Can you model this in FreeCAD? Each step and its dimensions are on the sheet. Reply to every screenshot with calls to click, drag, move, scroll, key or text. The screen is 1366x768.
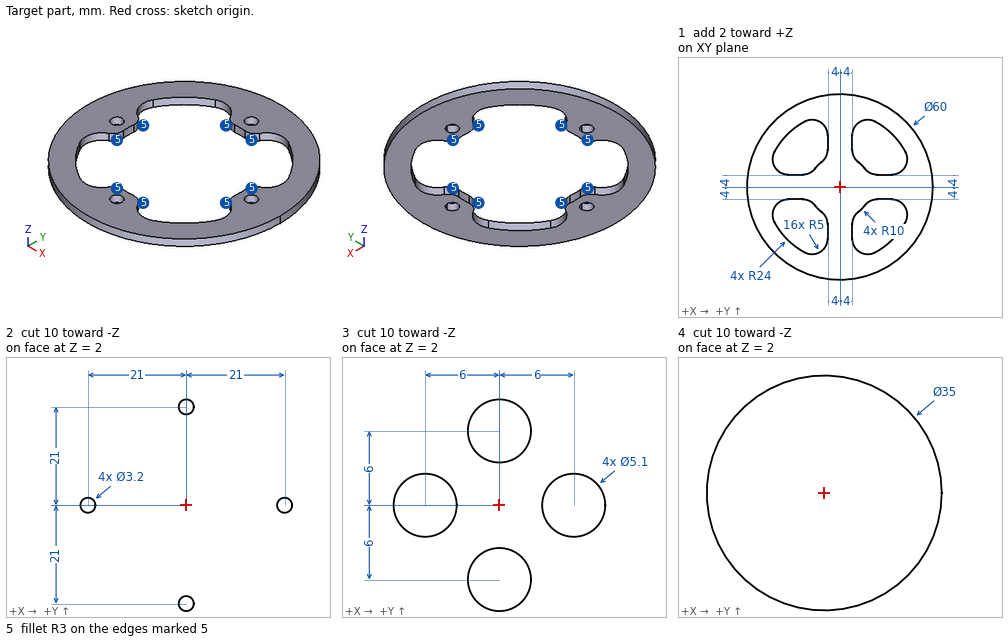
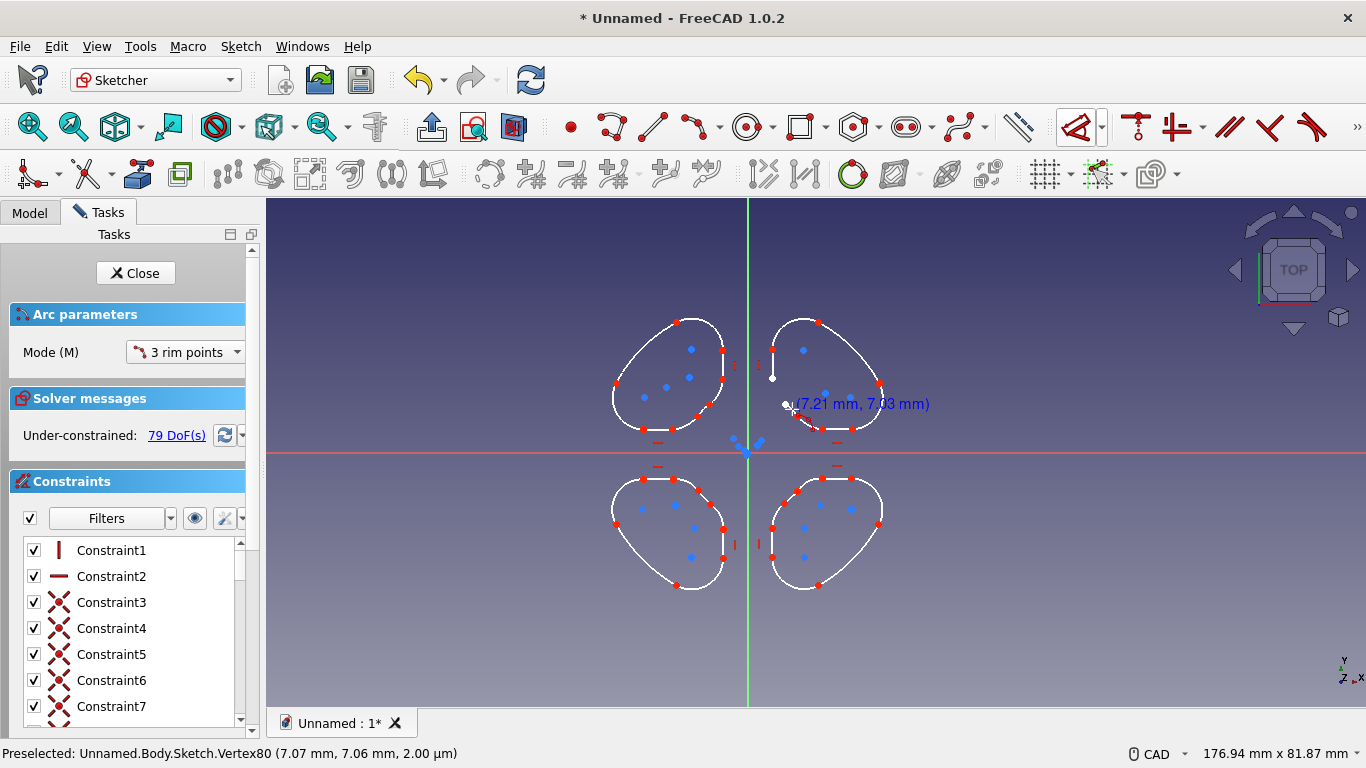
click(786, 404)
click(773, 379)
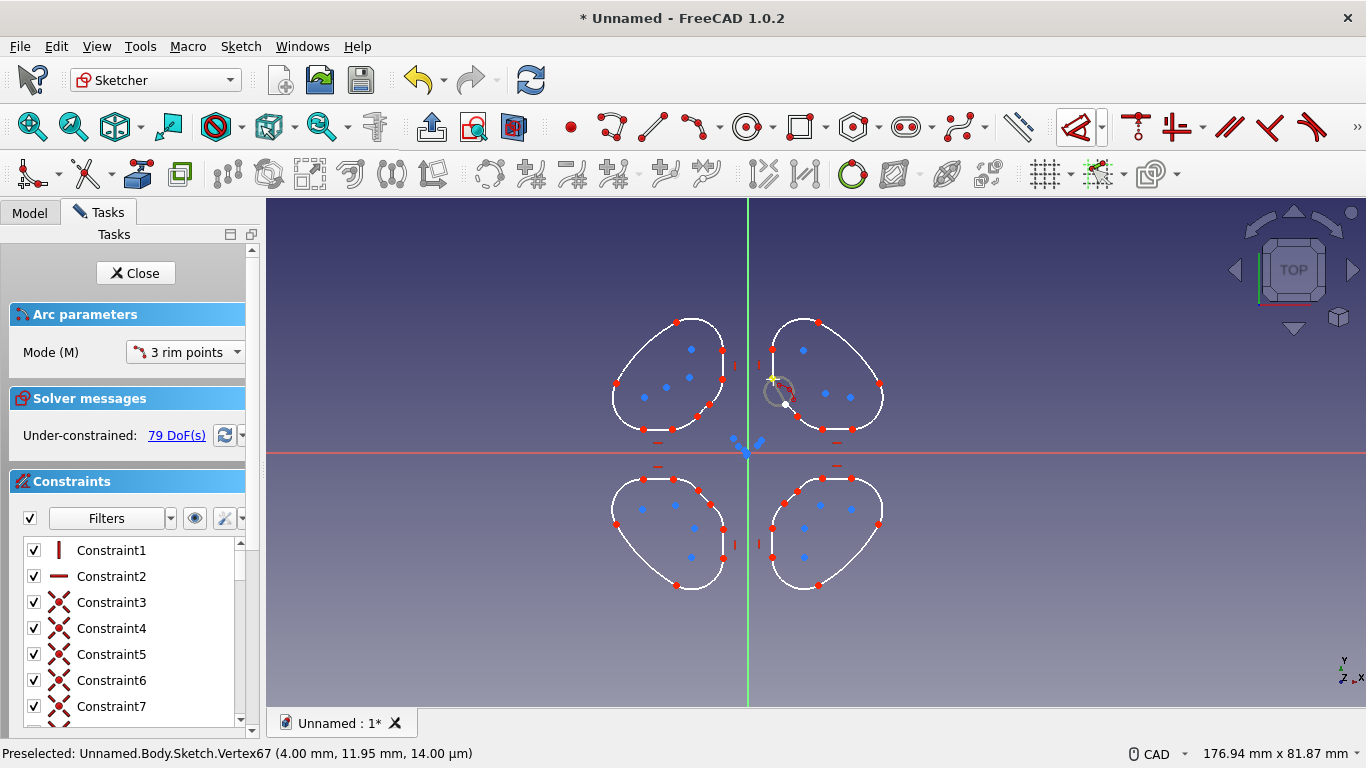
scroll(776, 392, up, 8)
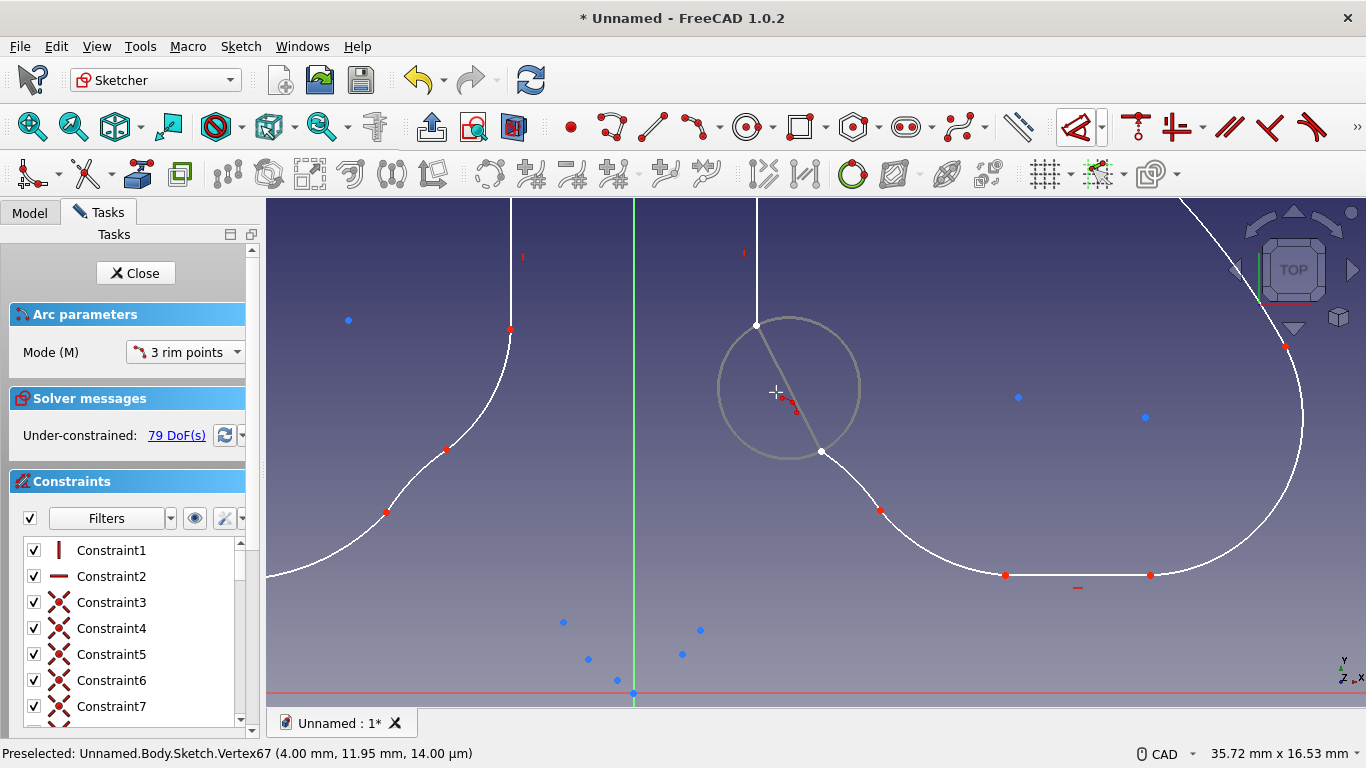
click(773, 393)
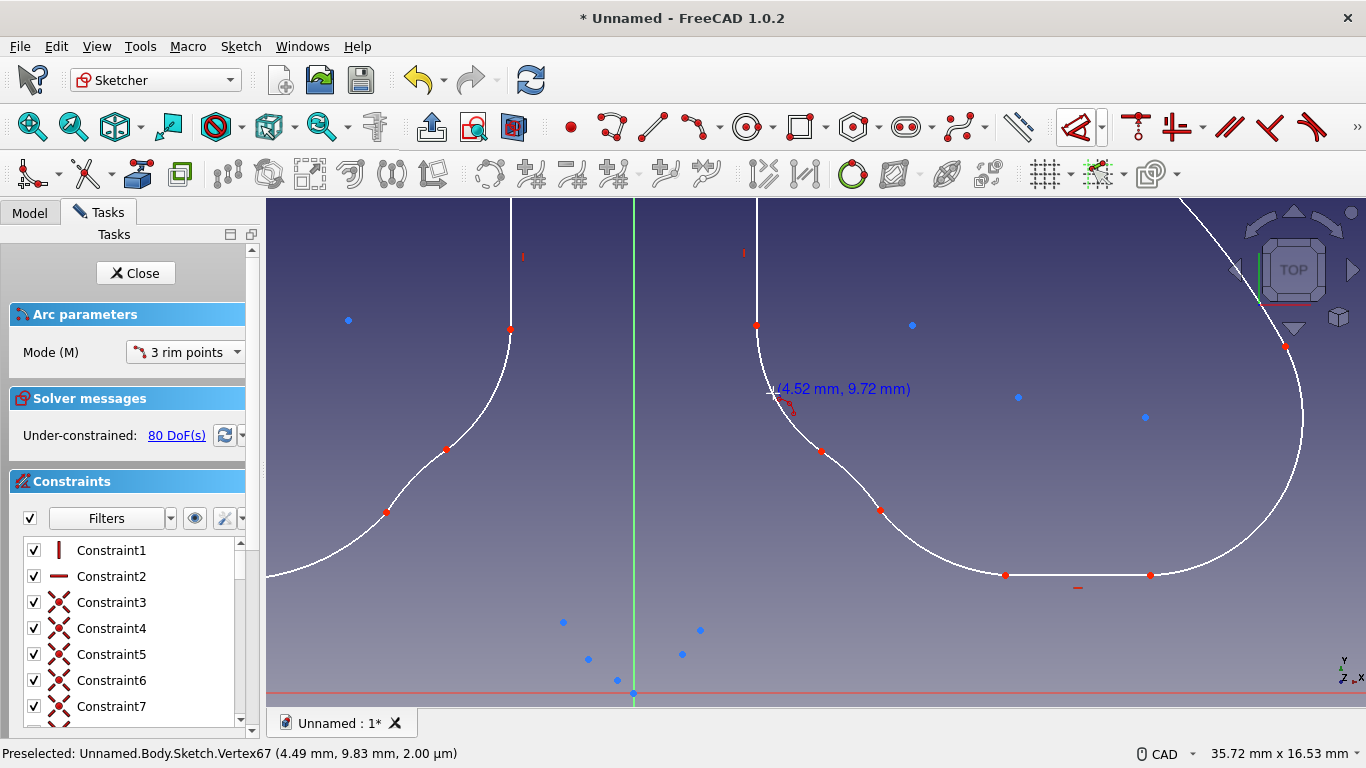
key(g)
key(c)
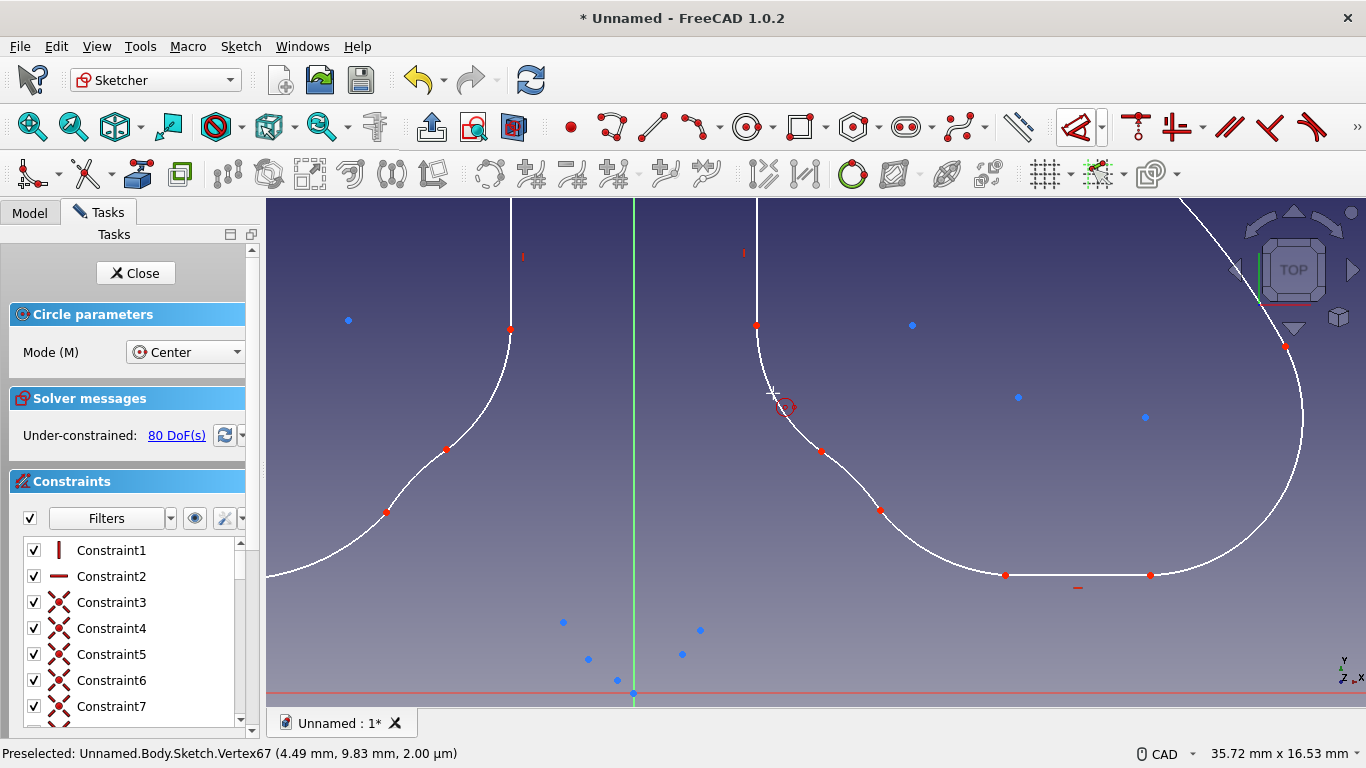
scroll(770, 405, down, 9)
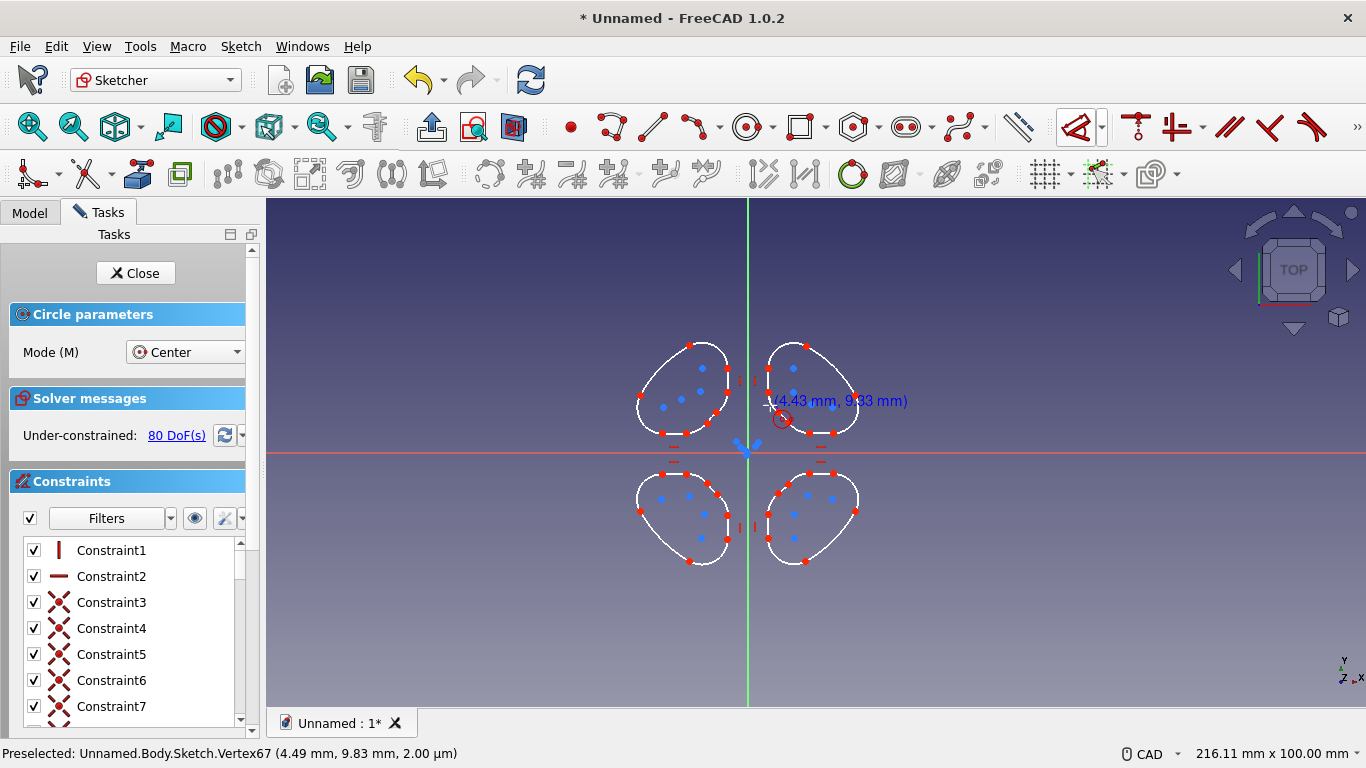
click(748, 453)
click(856, 345)
key(Escape)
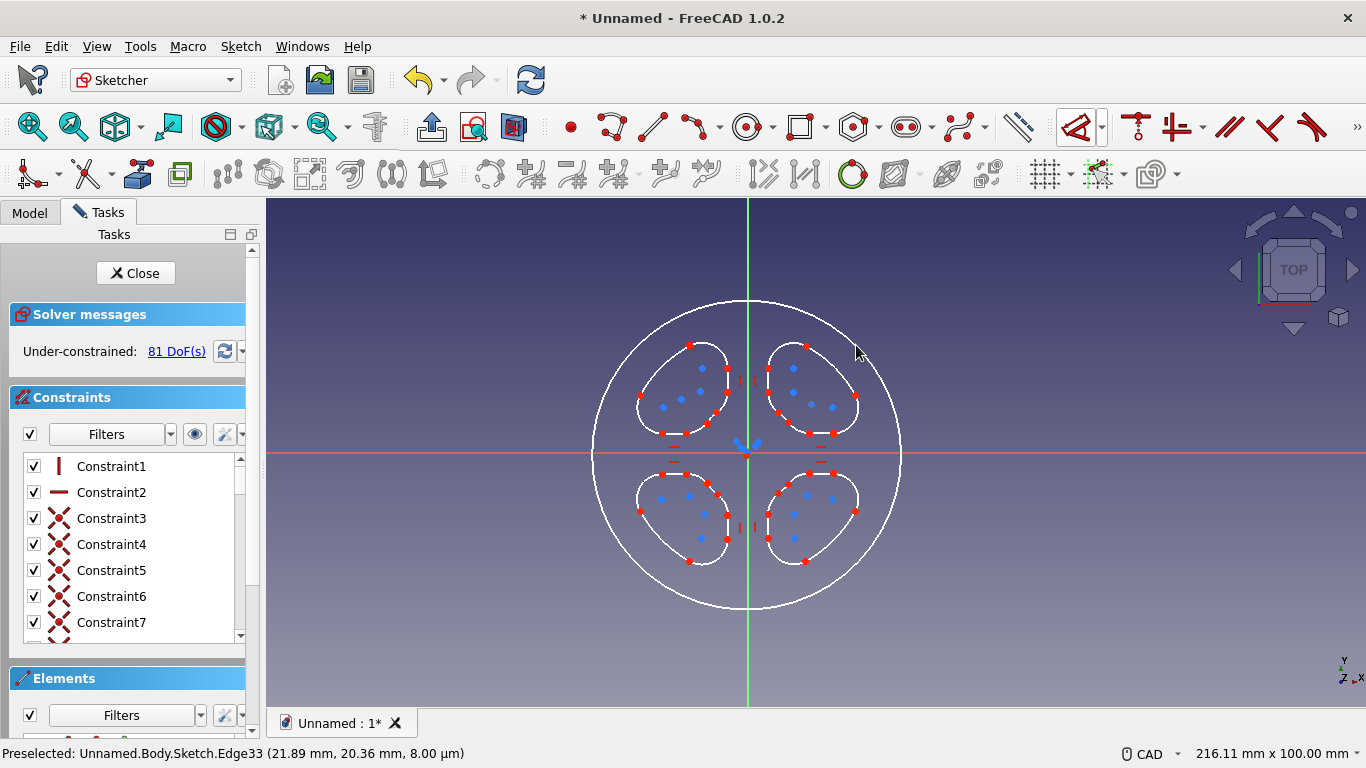
scroll(728, 525, up, 2)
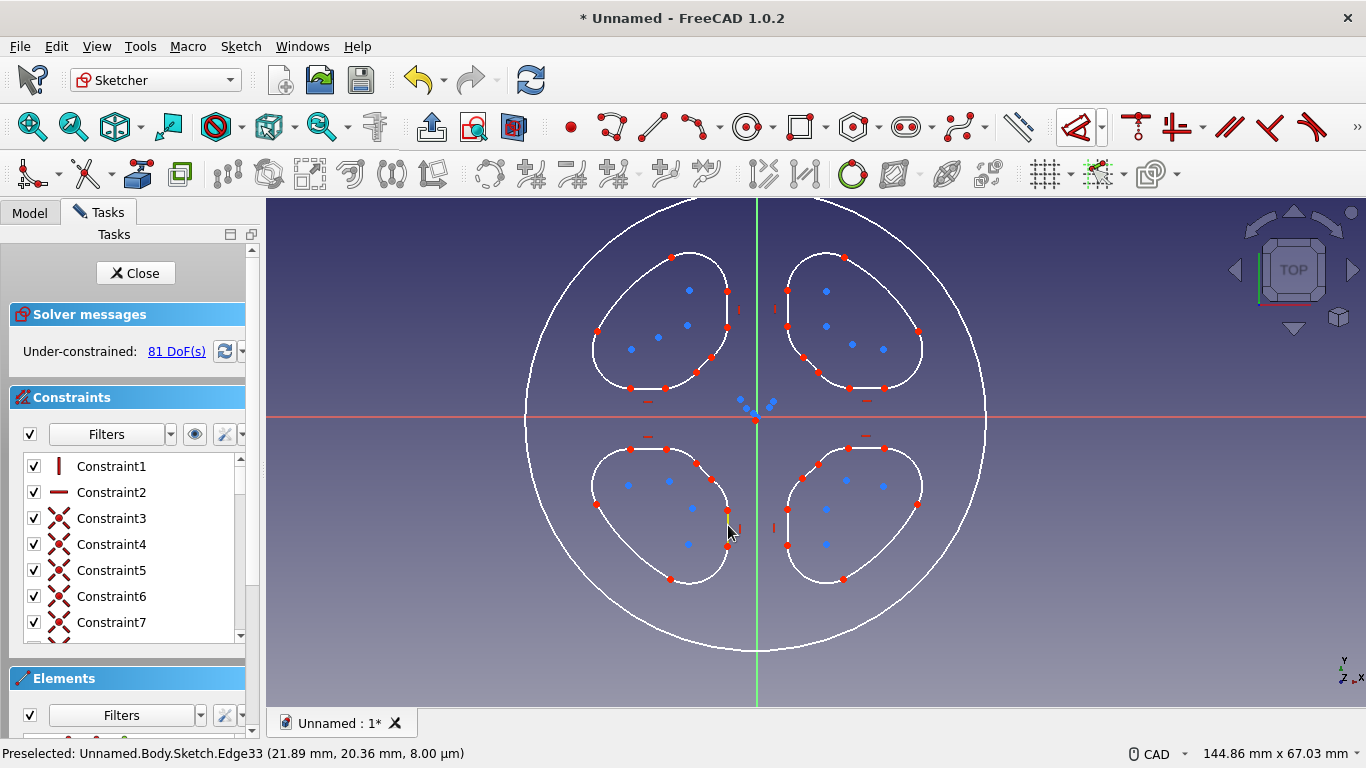
click(728, 525)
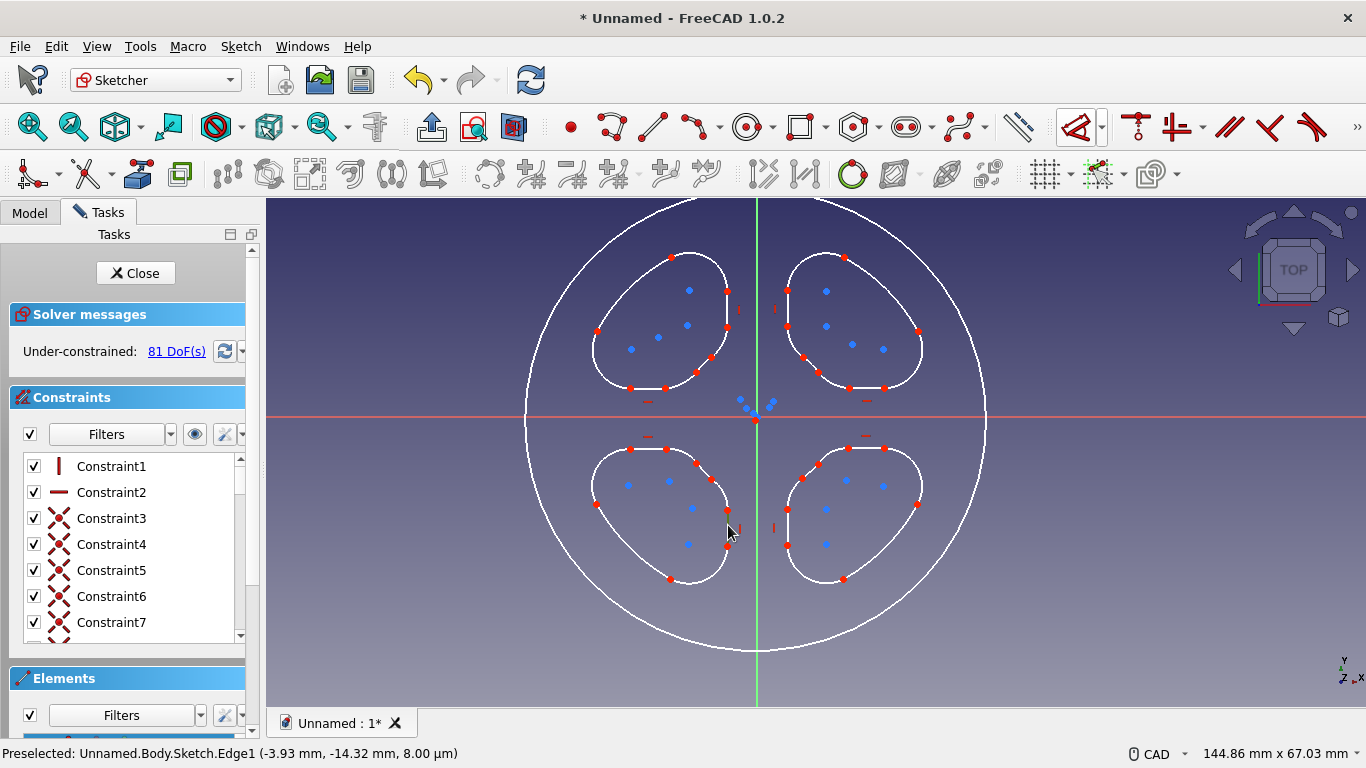
click(694, 583)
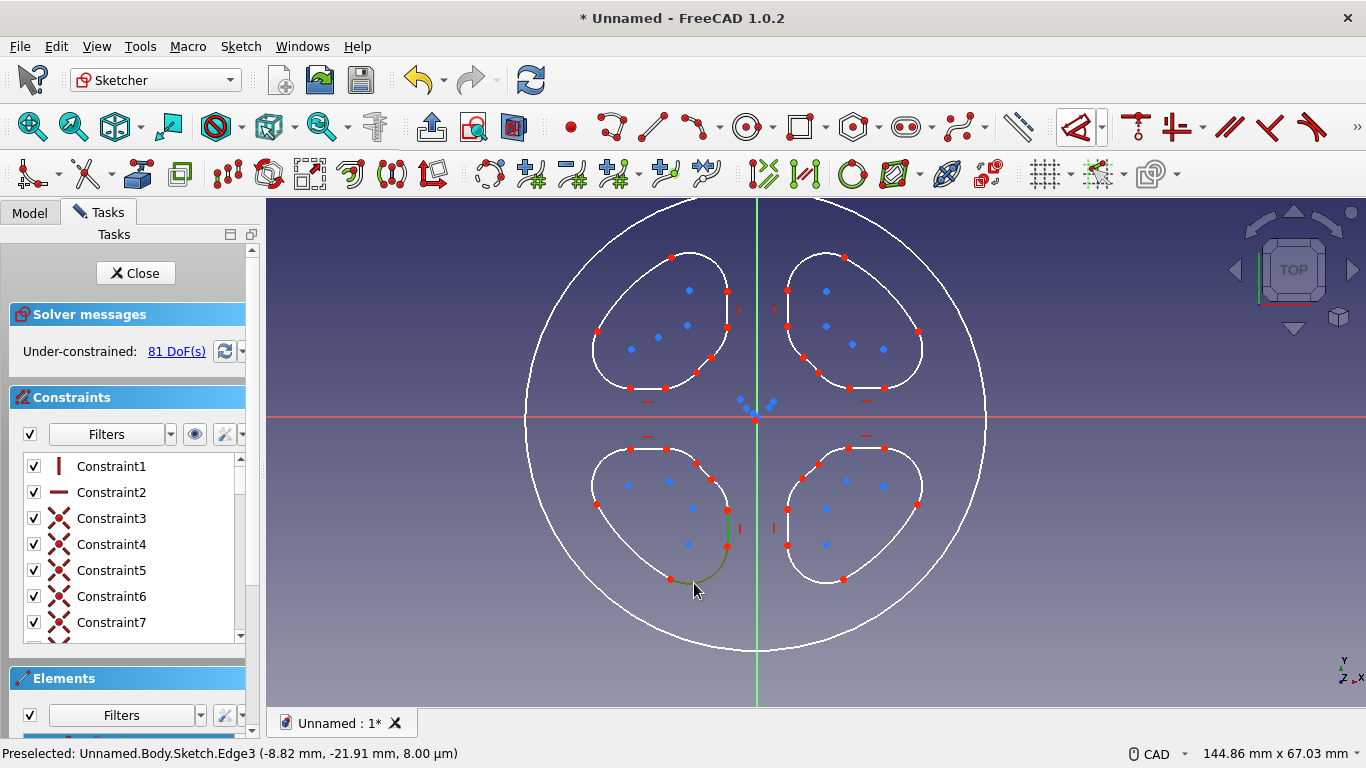
key(t)